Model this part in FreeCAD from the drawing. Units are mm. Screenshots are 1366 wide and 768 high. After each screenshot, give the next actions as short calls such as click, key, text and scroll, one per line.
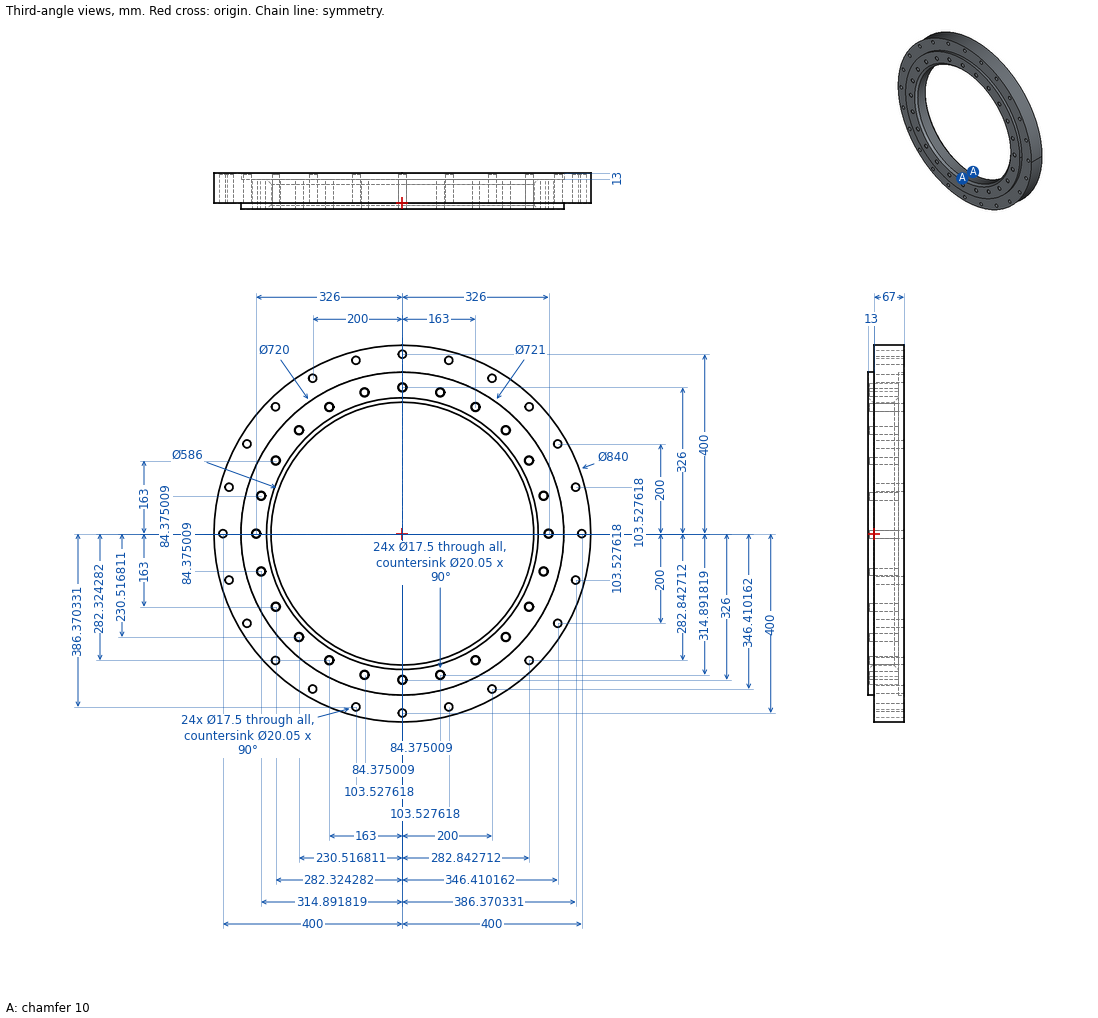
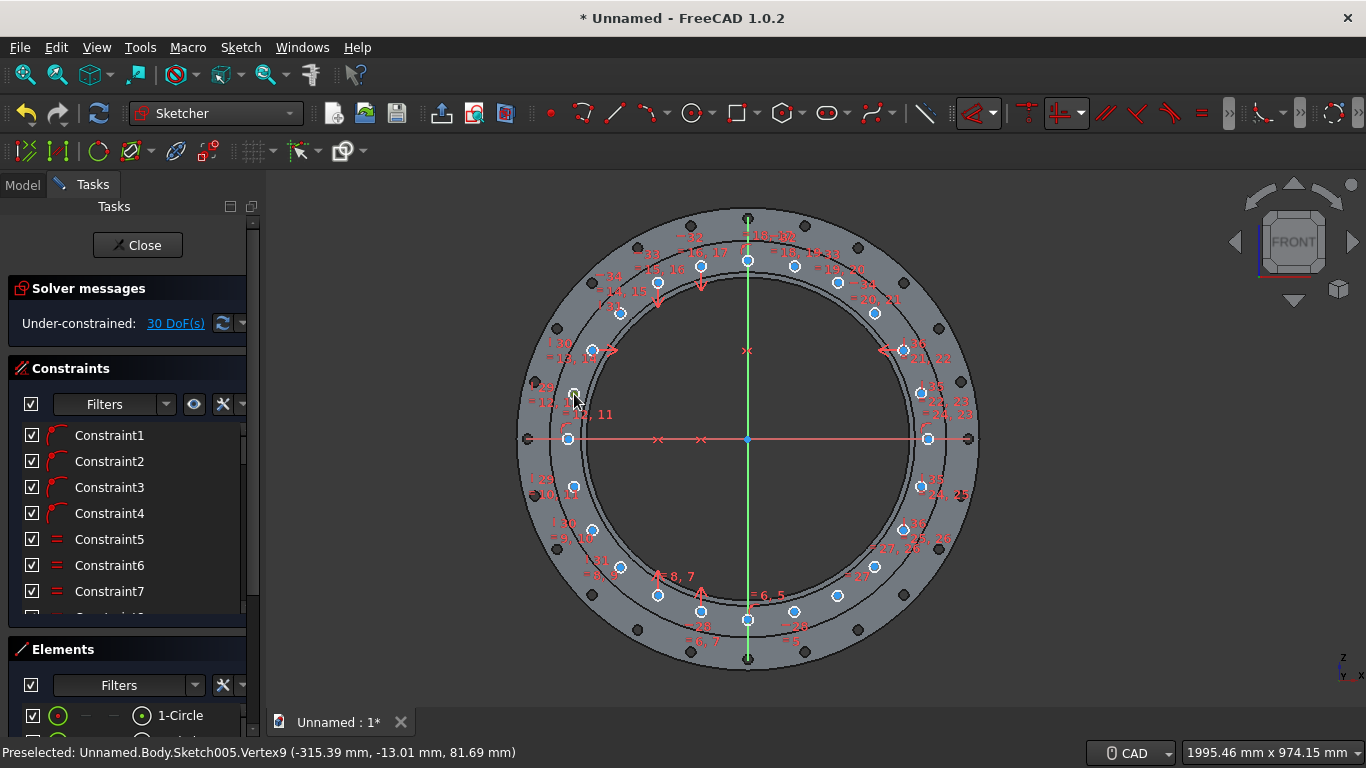
click(921, 393)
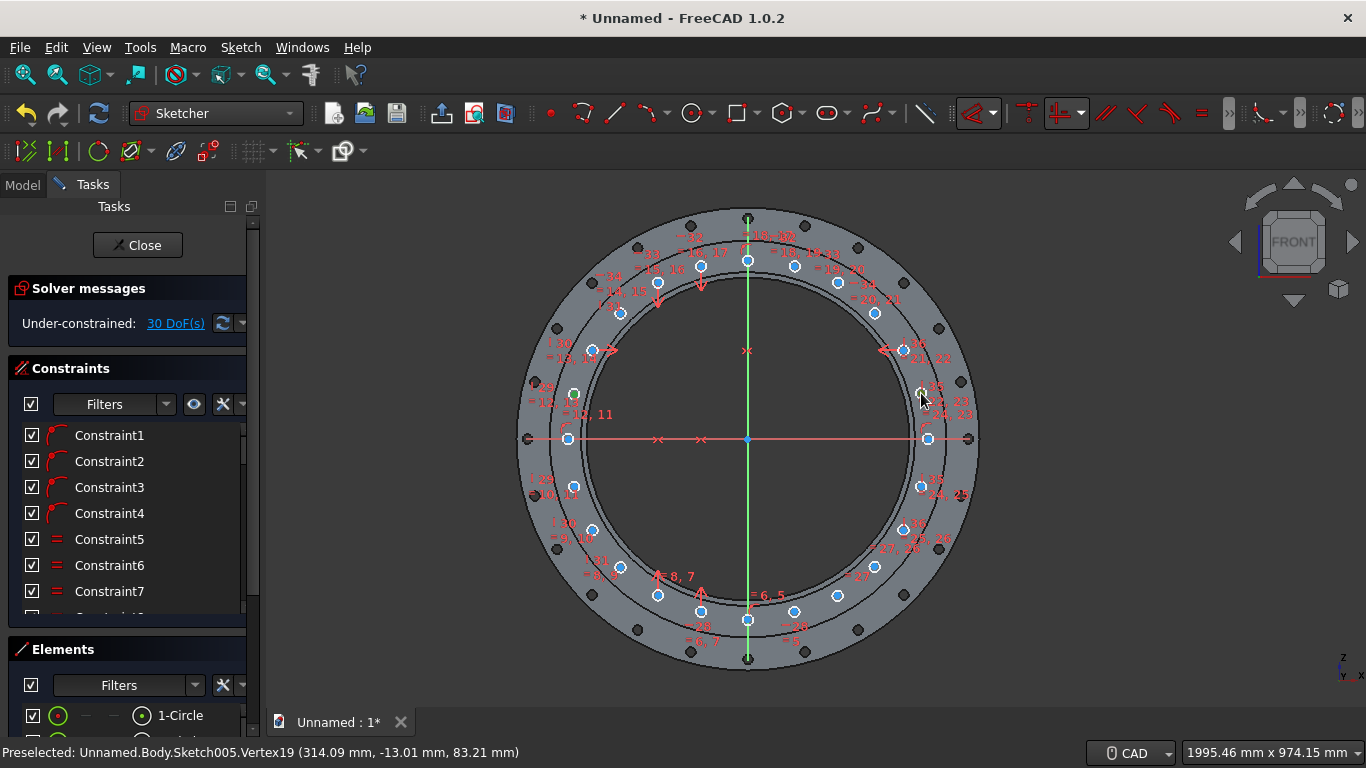
click(748, 576)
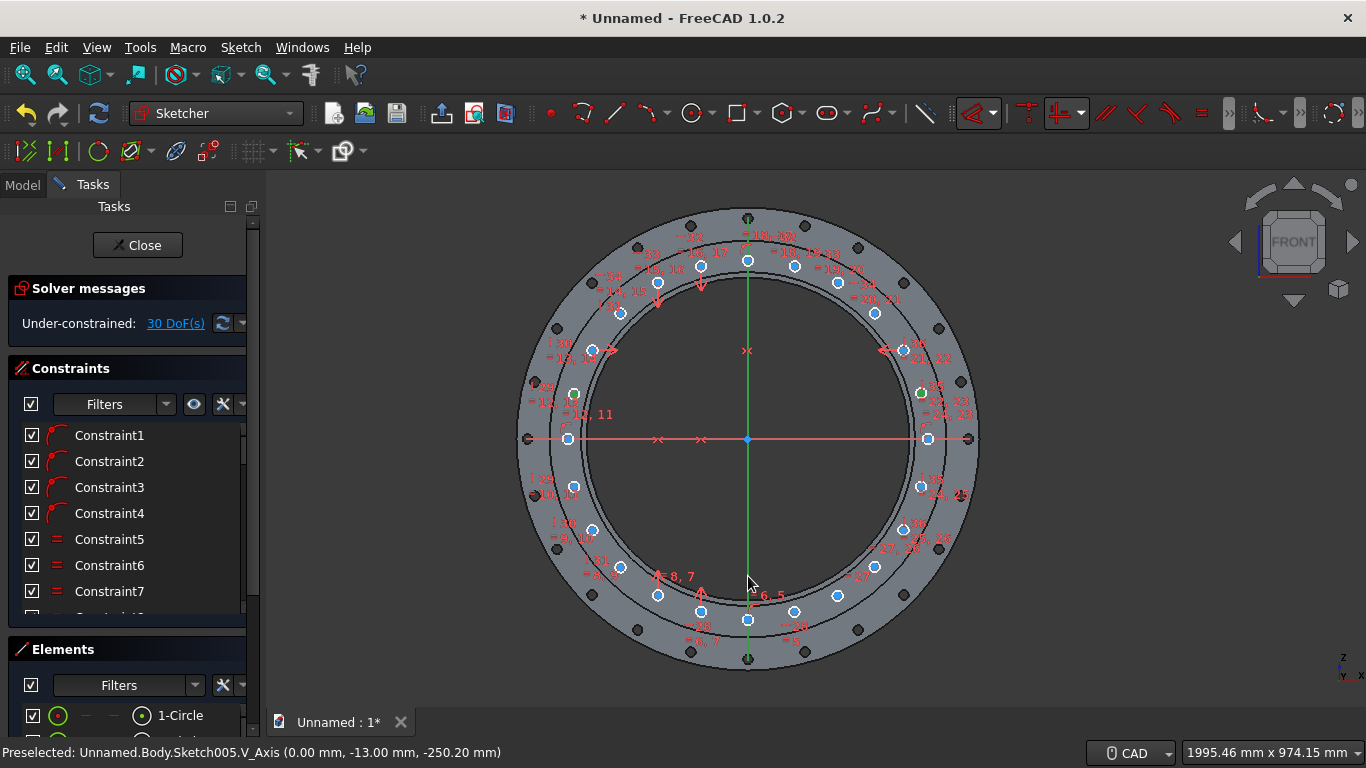
key(s)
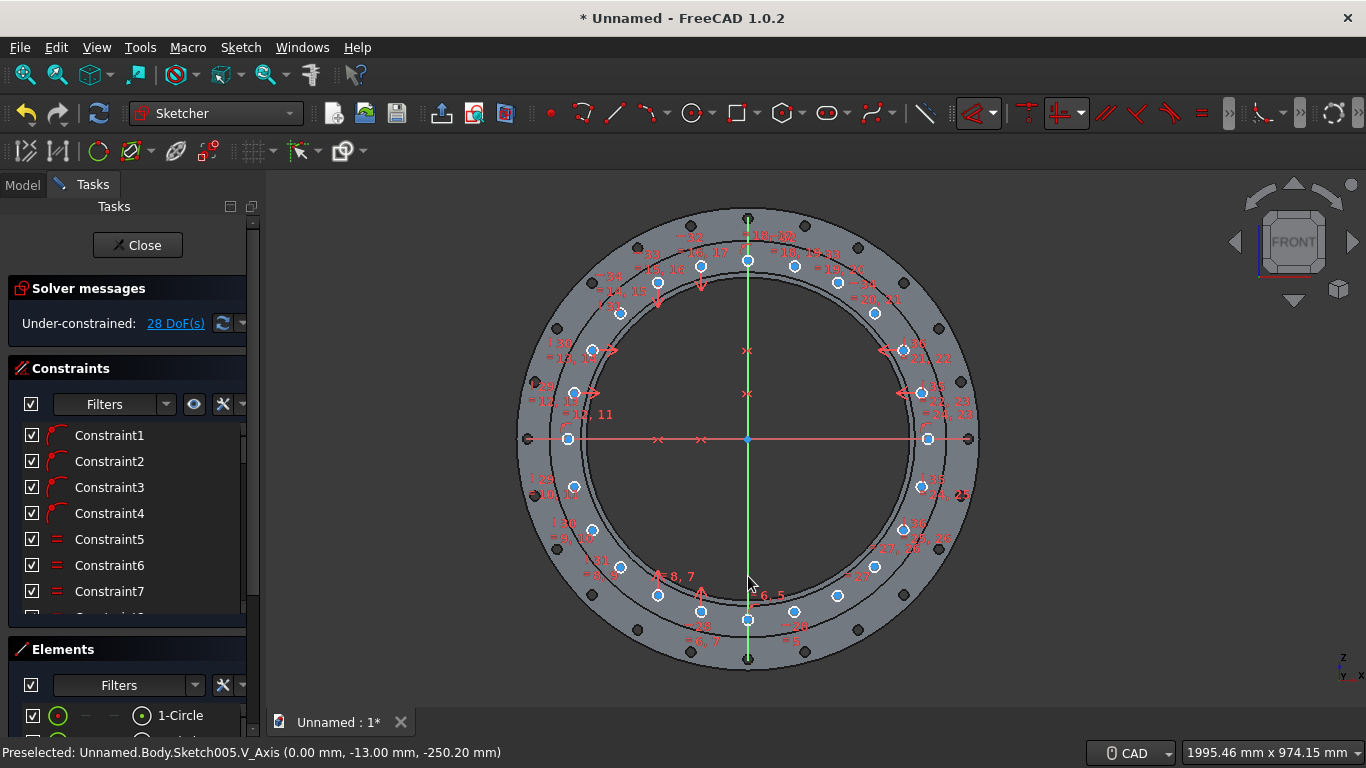
click(621, 567)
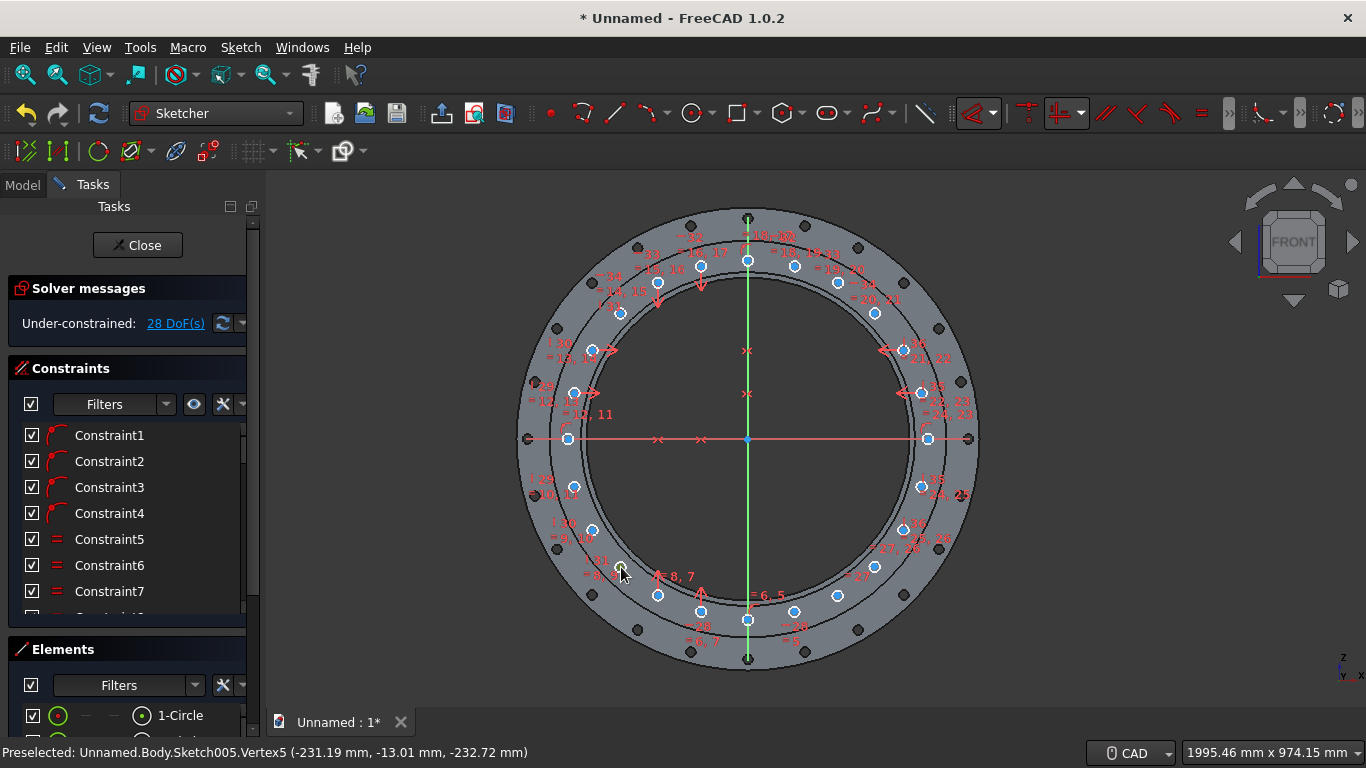
click(875, 567)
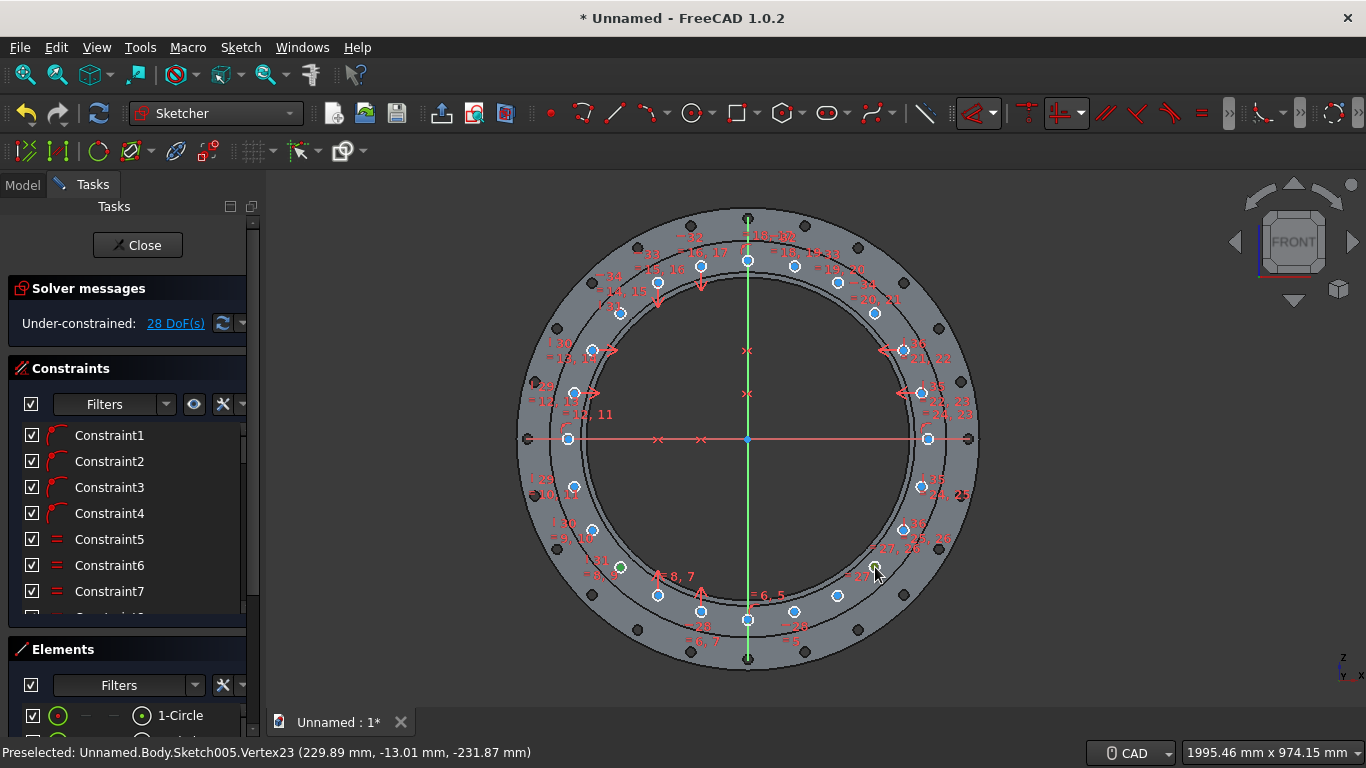
click(748, 576)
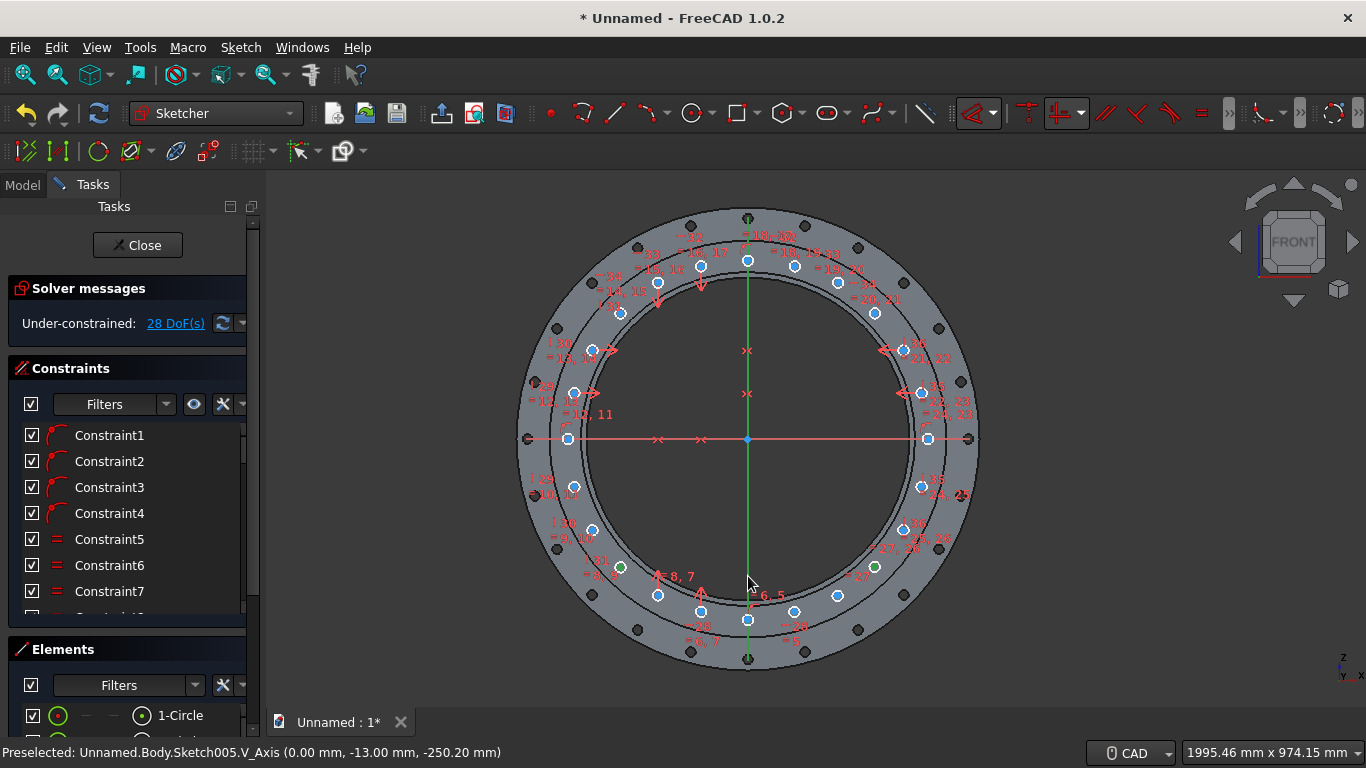
key(s)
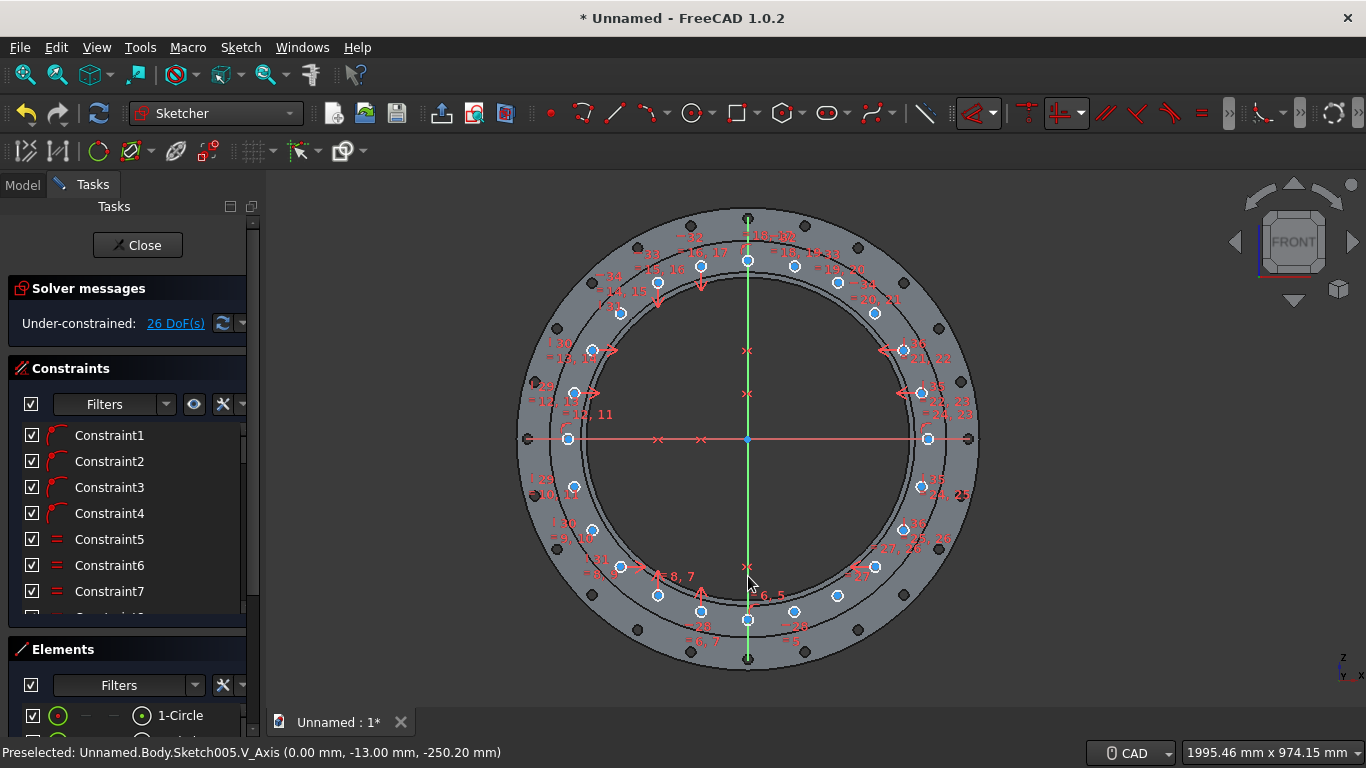
click(875, 313)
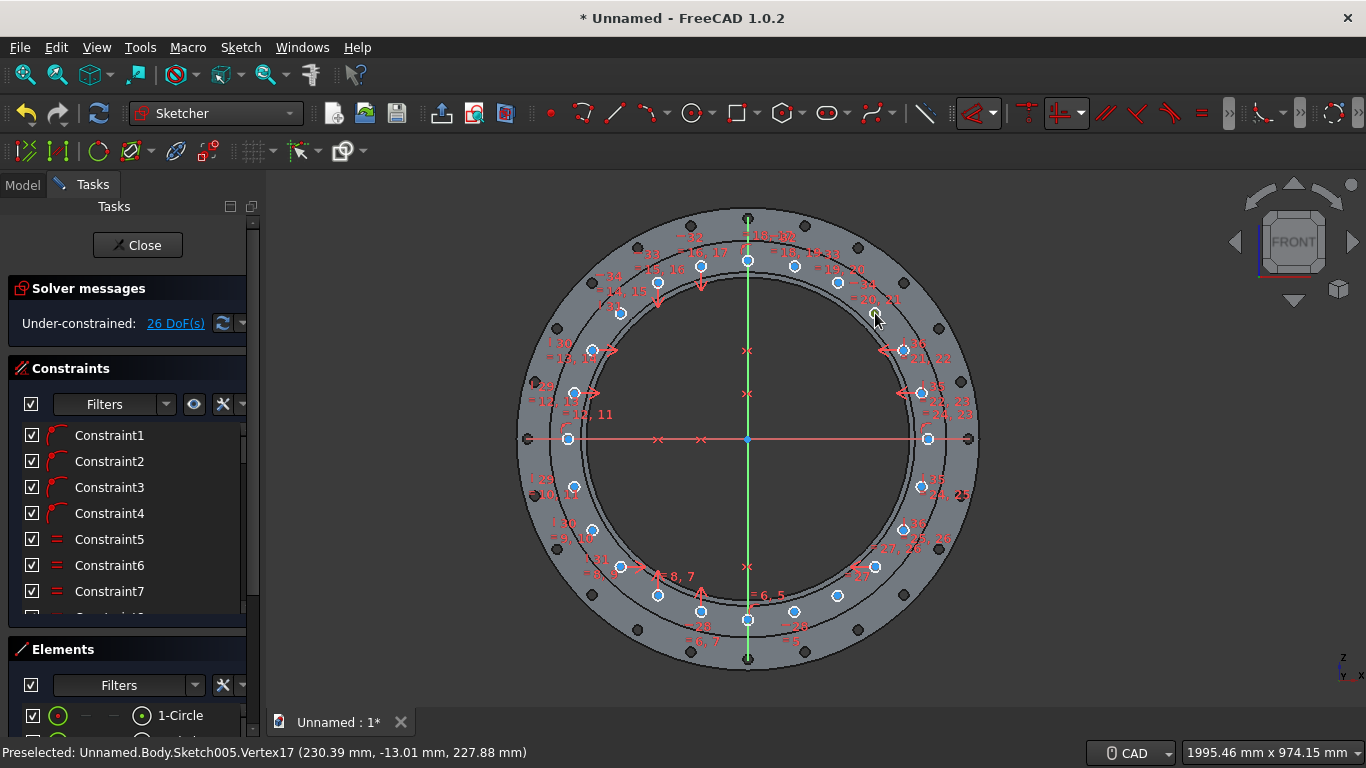
click(875, 567)